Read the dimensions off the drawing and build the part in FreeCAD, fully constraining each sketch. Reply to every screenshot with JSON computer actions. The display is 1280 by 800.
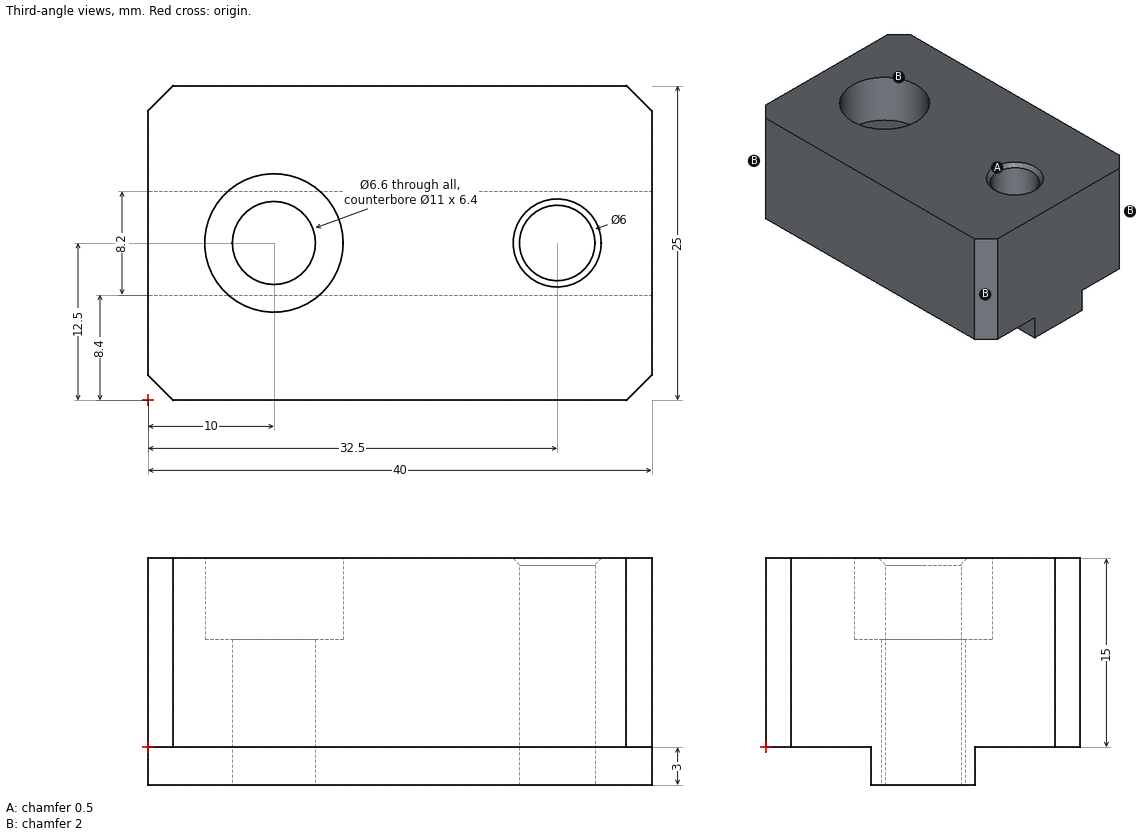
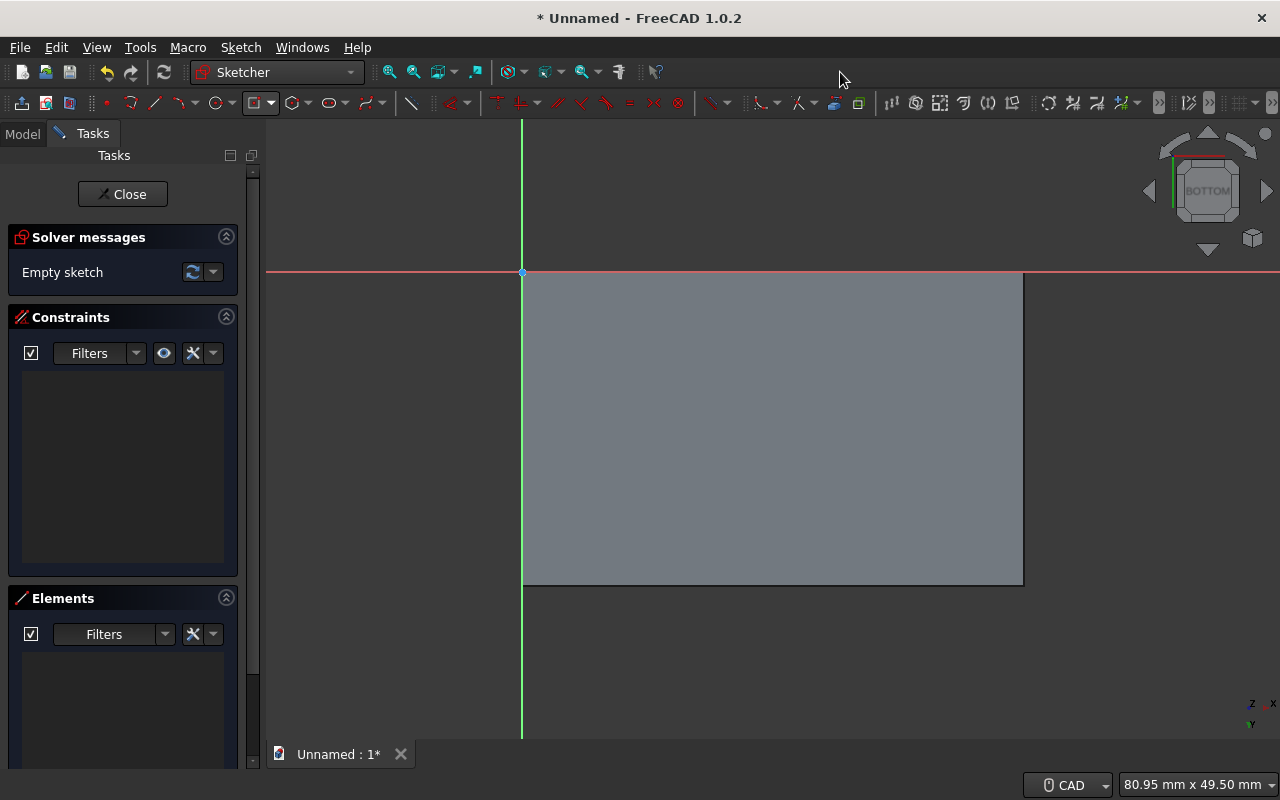
{"action": "key", "text": "g r"}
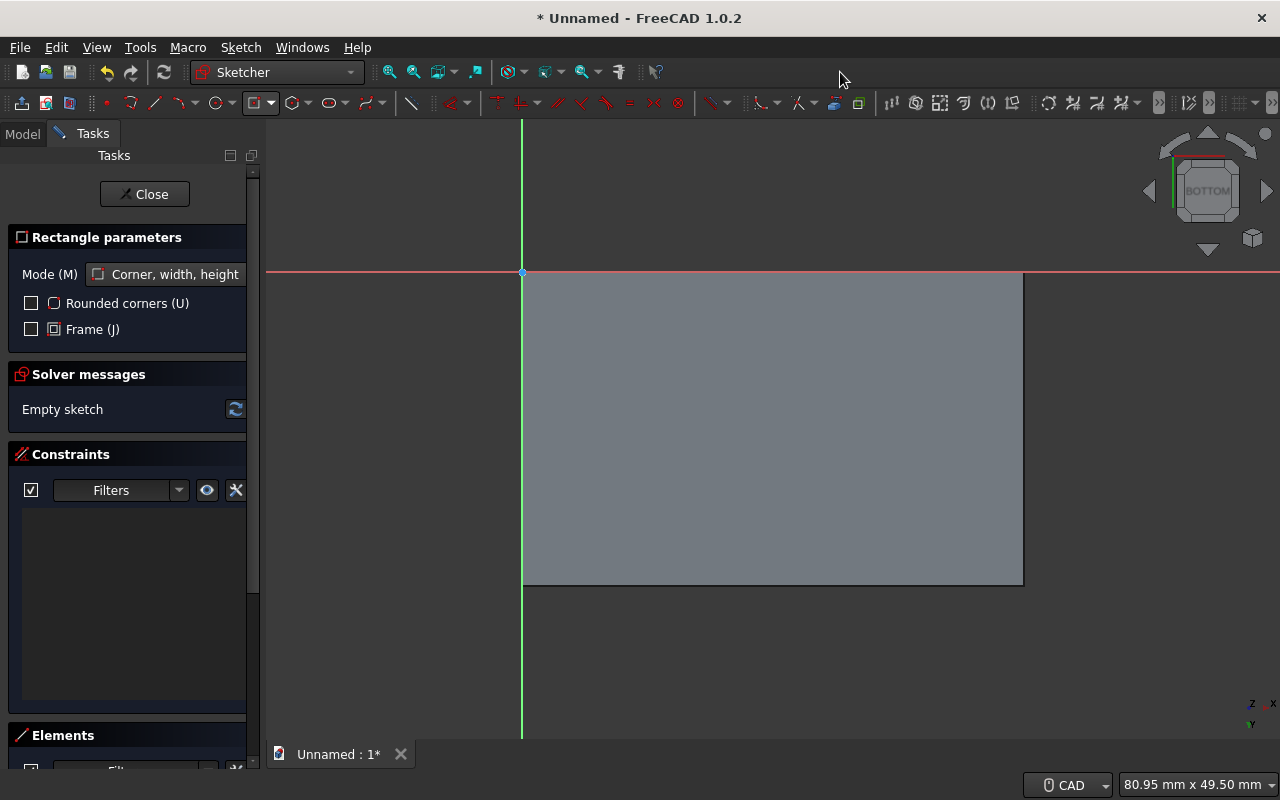
{"action": "left_click", "coordinate": [522, 378]}
{"action": "left_click", "coordinate": [1024, 480]}
{"action": "key", "text": "Escape"}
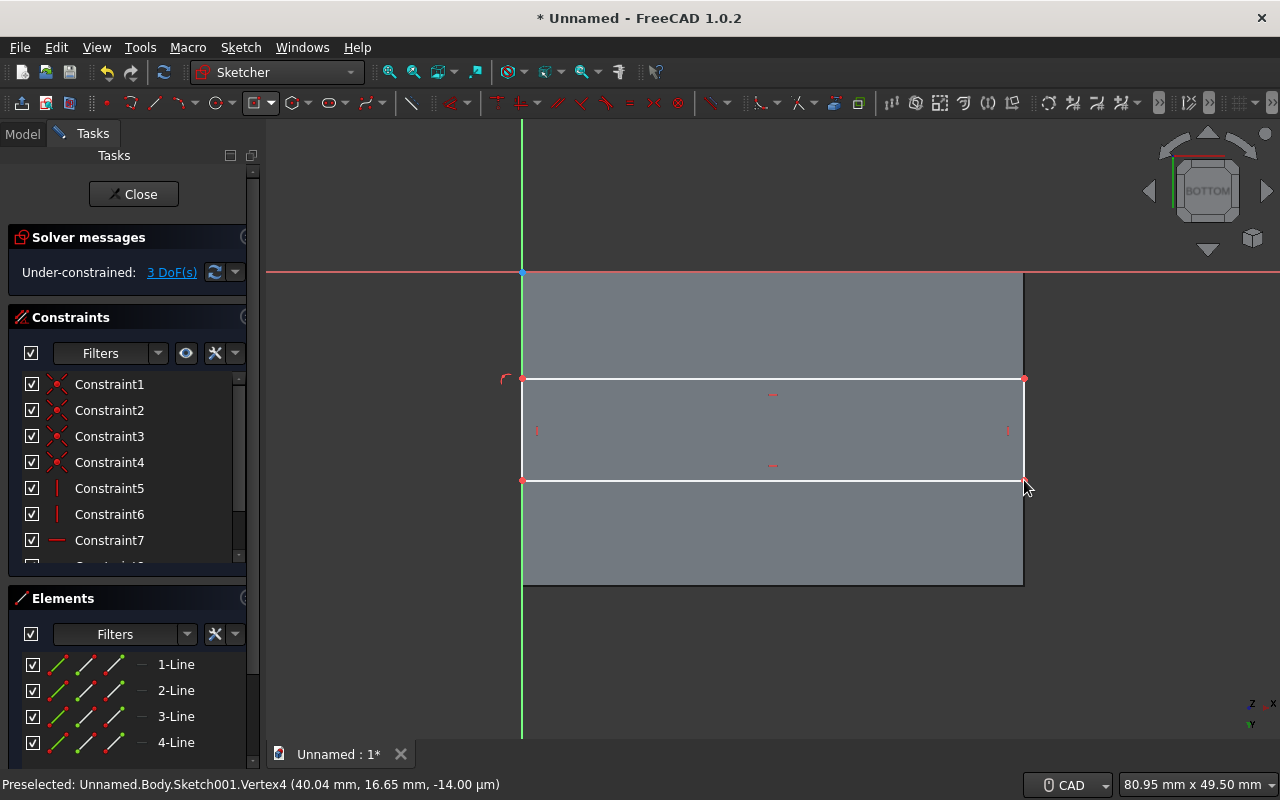
{"action": "left_click", "coordinate": [450, 104]}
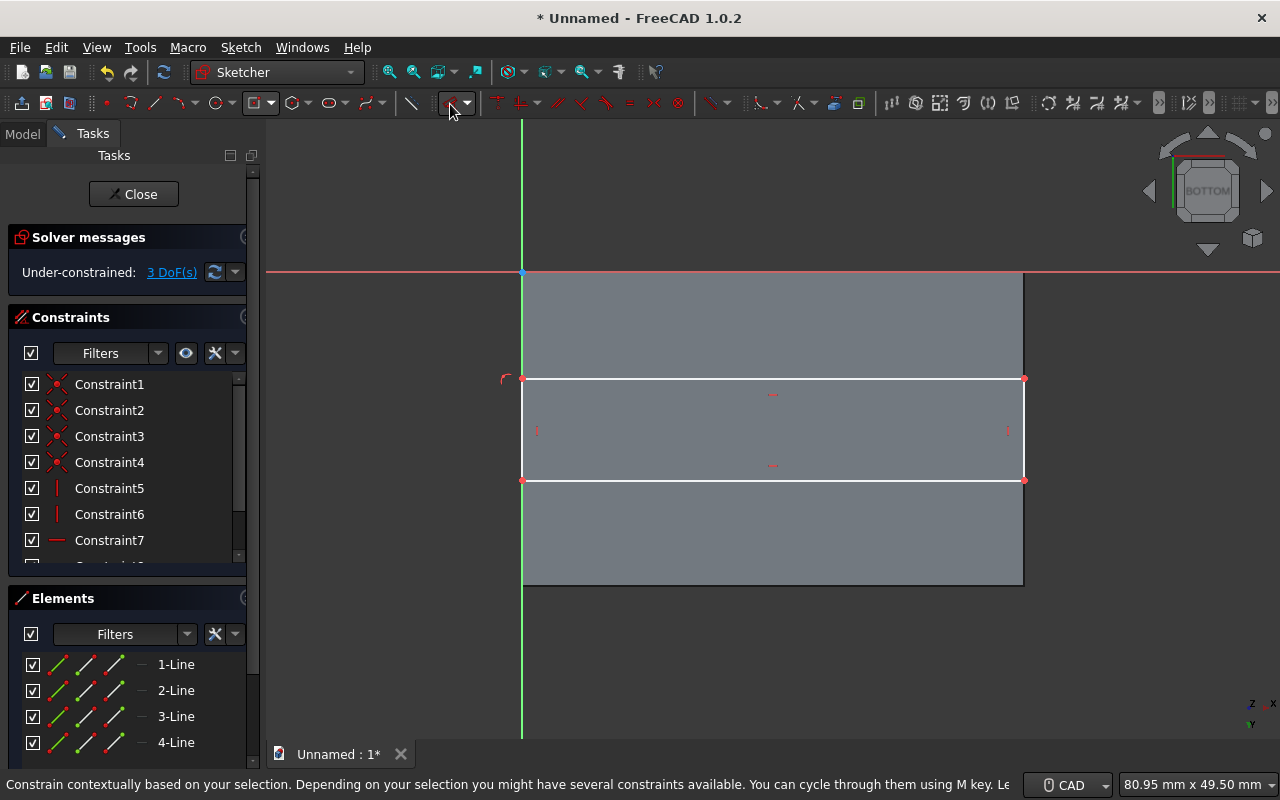
{"action": "left_click", "coordinate": [673, 481]}
{"action": "left_click", "coordinate": [773, 515]}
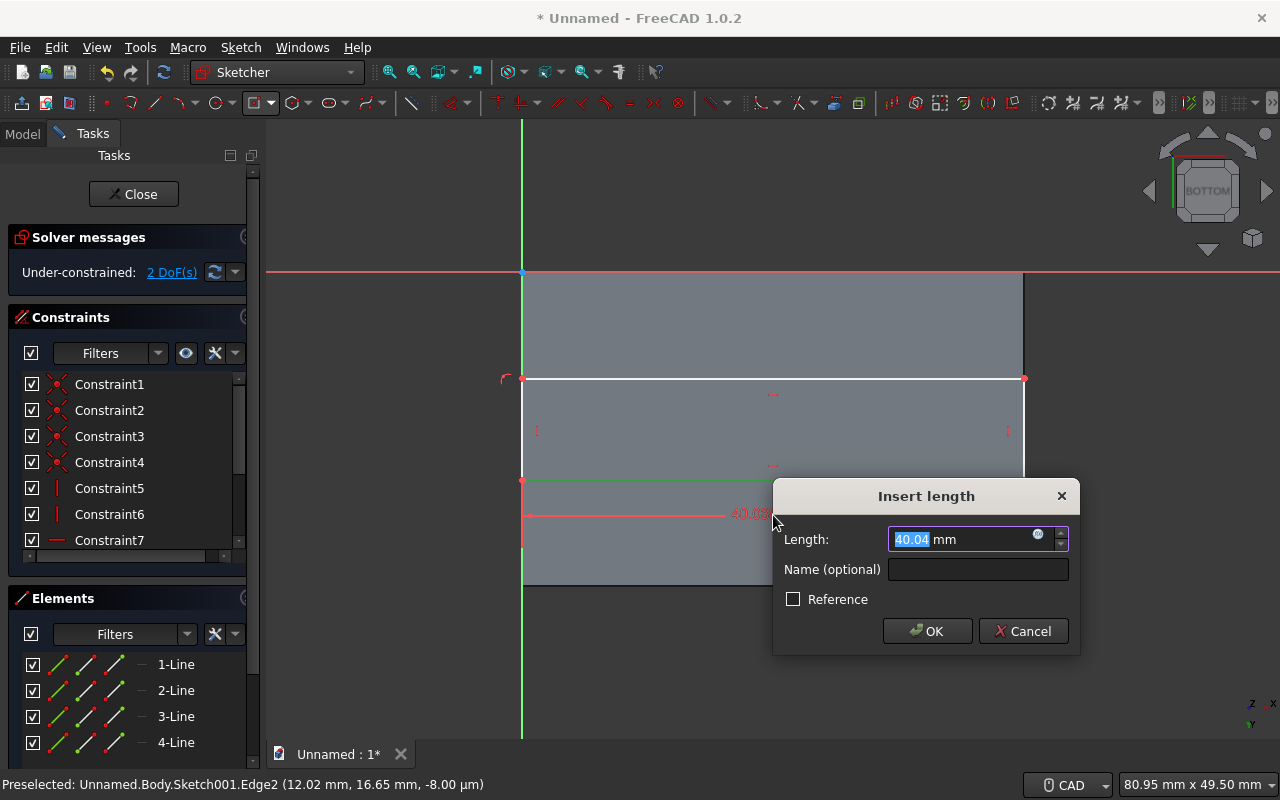
{"action": "type", "text": "40"}
{"action": "key", "text": "Return"}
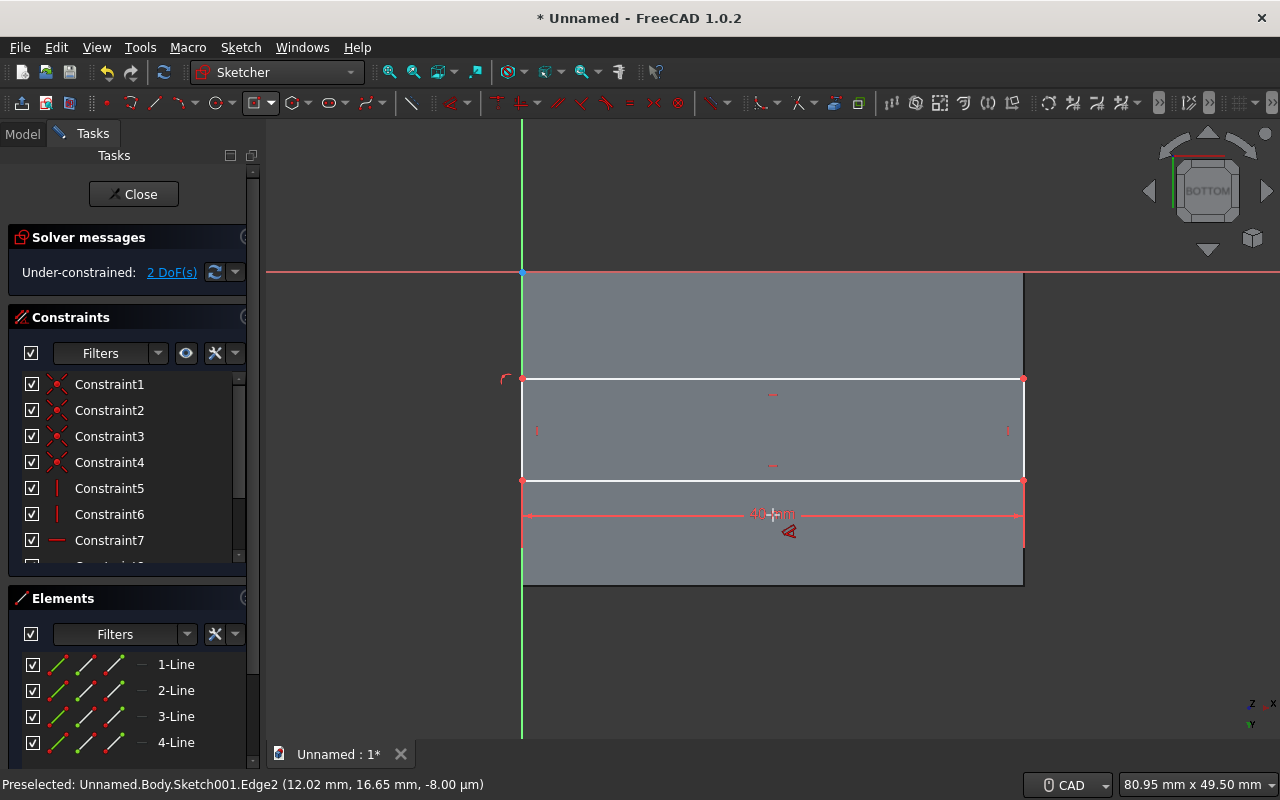
{"action": "left_click", "coordinate": [522, 410]}
{"action": "left_click", "coordinate": [488, 430]}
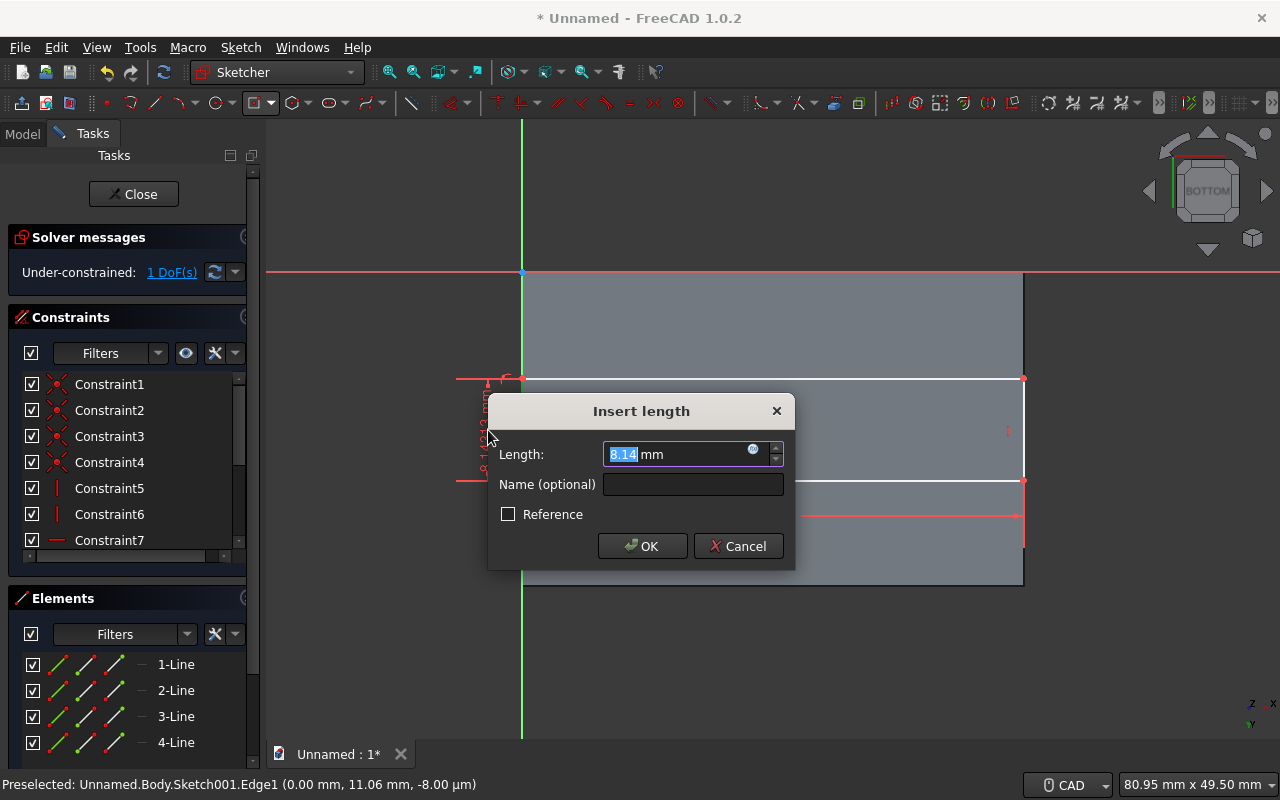
{"action": "type", "text": "8.2"}
{"action": "key", "text": "Return"}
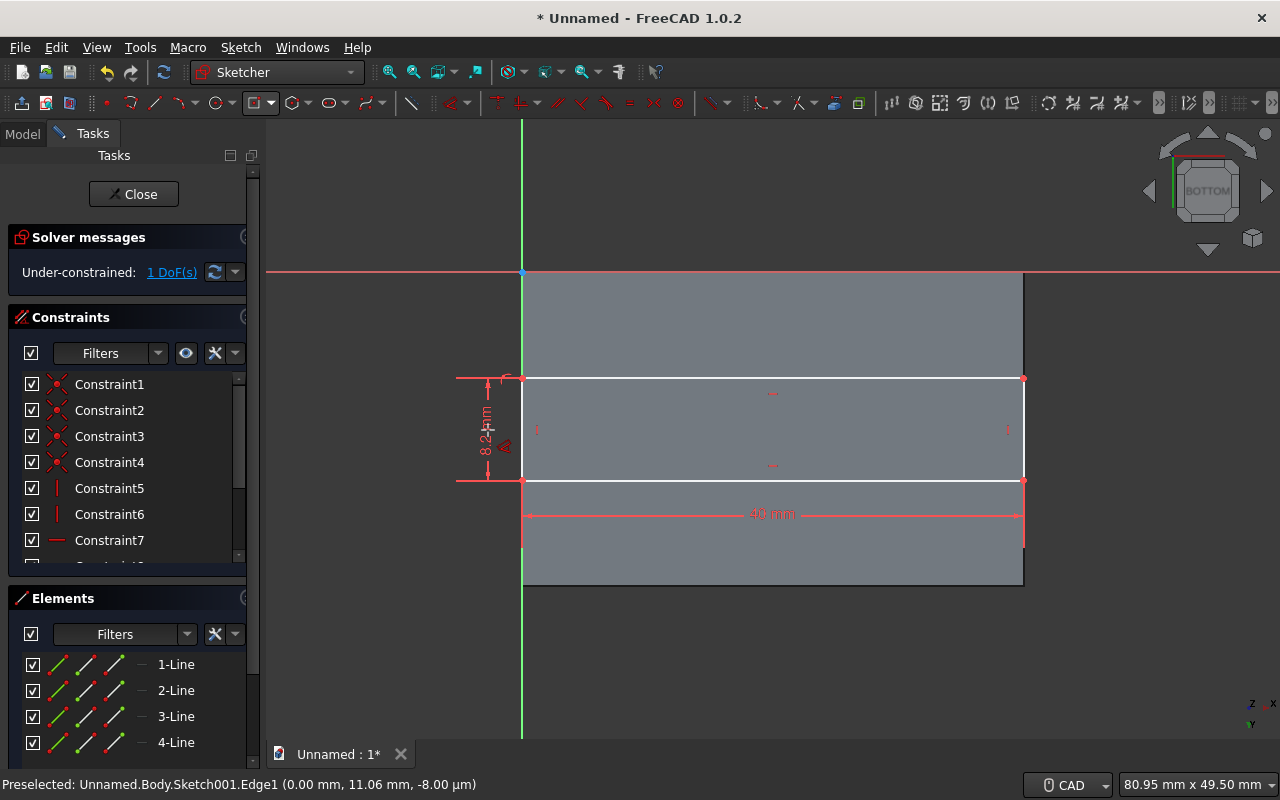
{"action": "left_click", "coordinate": [522, 378]}
{"action": "left_click", "coordinate": [488, 325]}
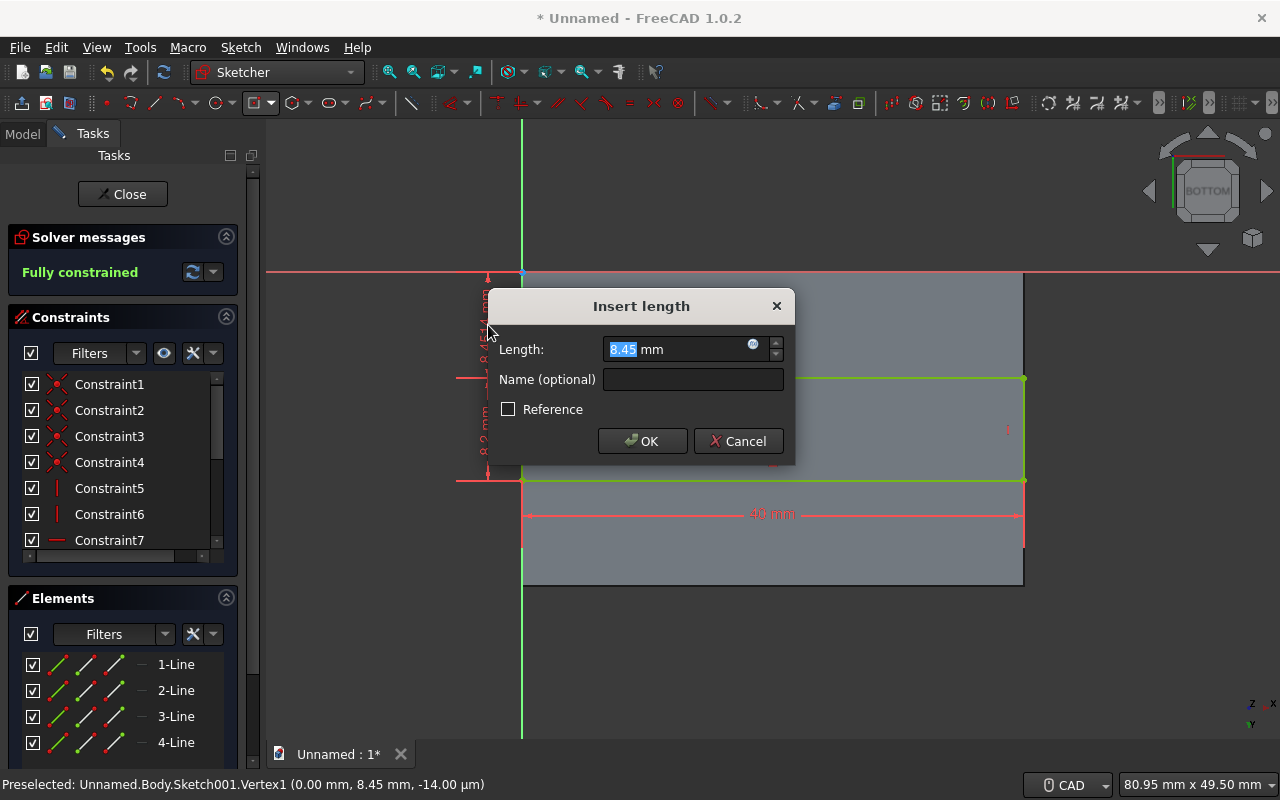
{"action": "type", "text": "8.4"}
{"action": "key", "text": "Return"}
{"action": "key", "text": "Escape"}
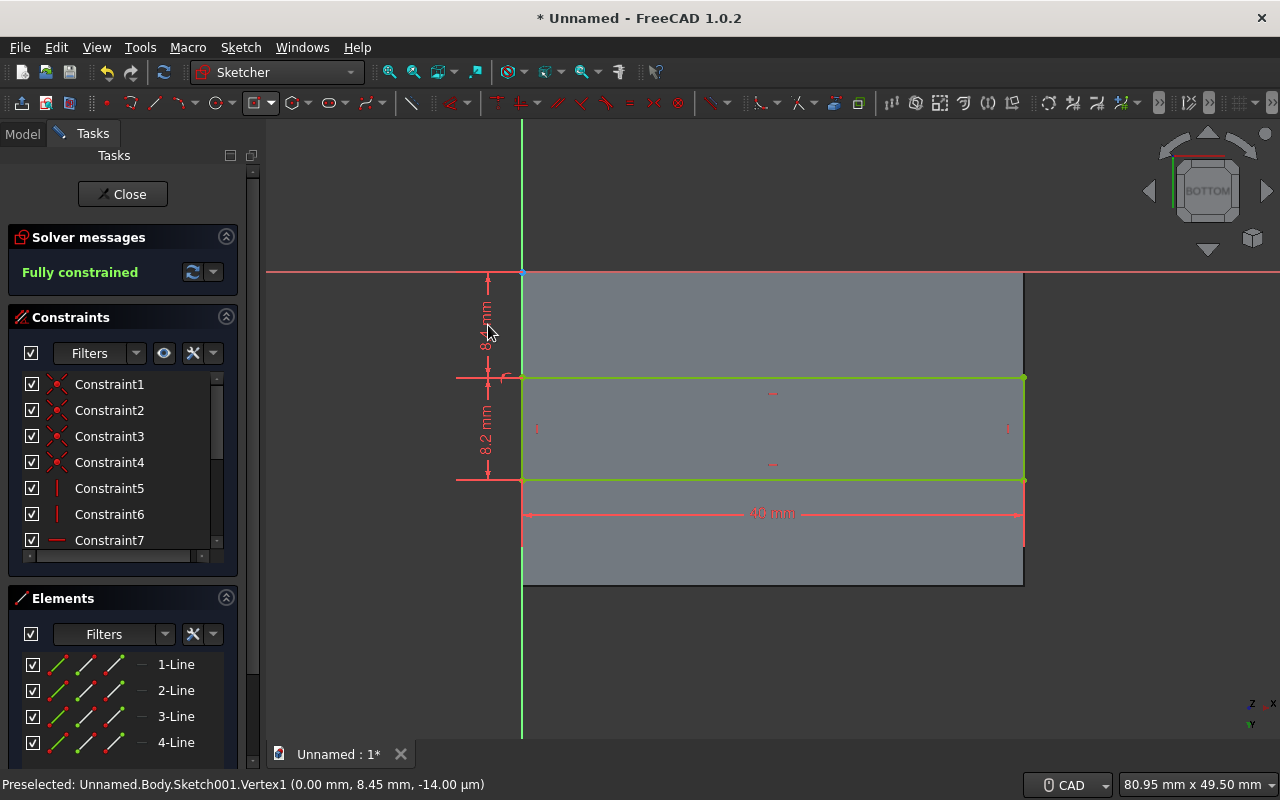
{"action": "left_click", "coordinate": [123, 194]}